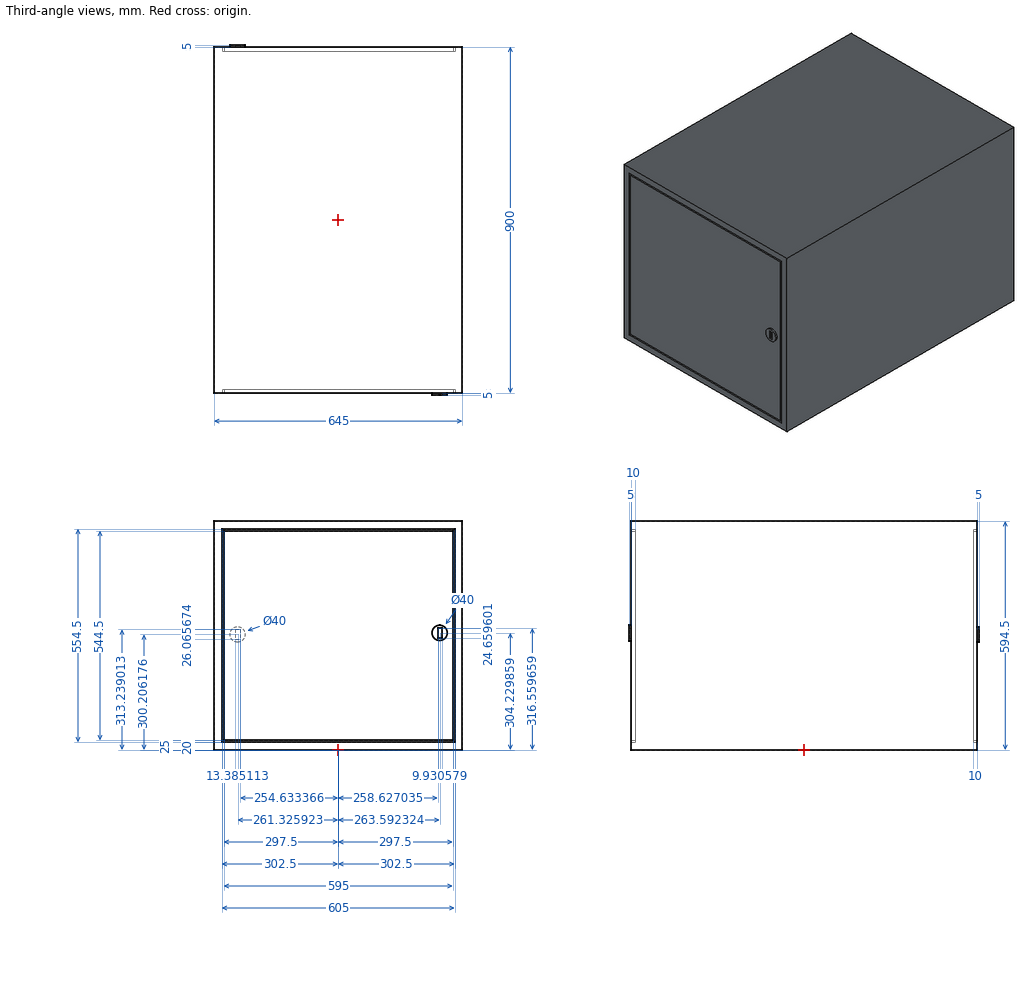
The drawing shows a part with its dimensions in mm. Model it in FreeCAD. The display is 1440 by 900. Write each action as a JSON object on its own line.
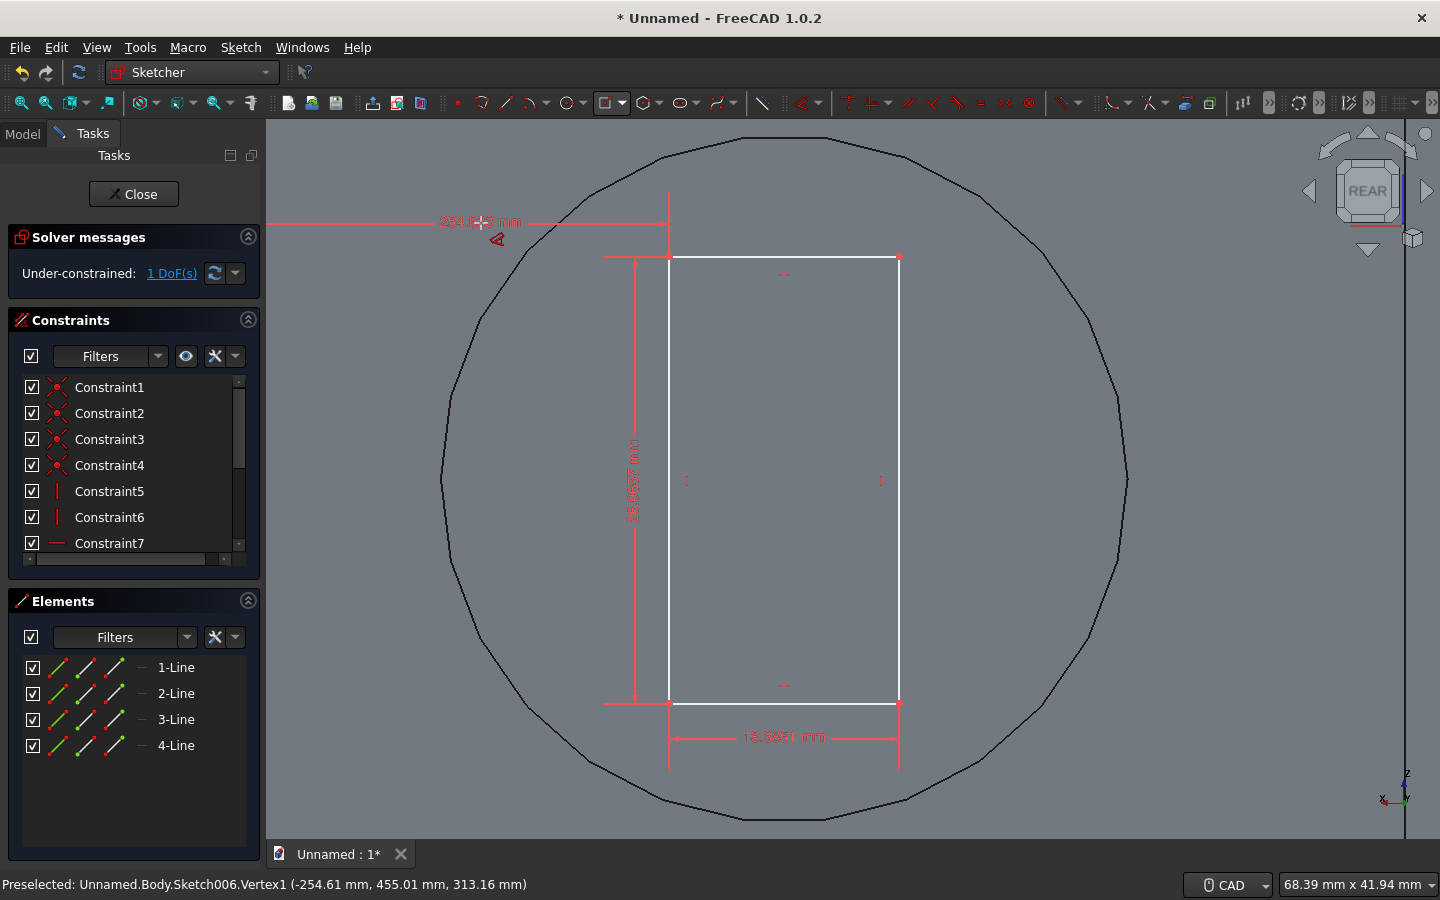
{"action": "left_click", "coordinate": [669, 257]}
{"action": "left_click", "coordinate": [703, 534]}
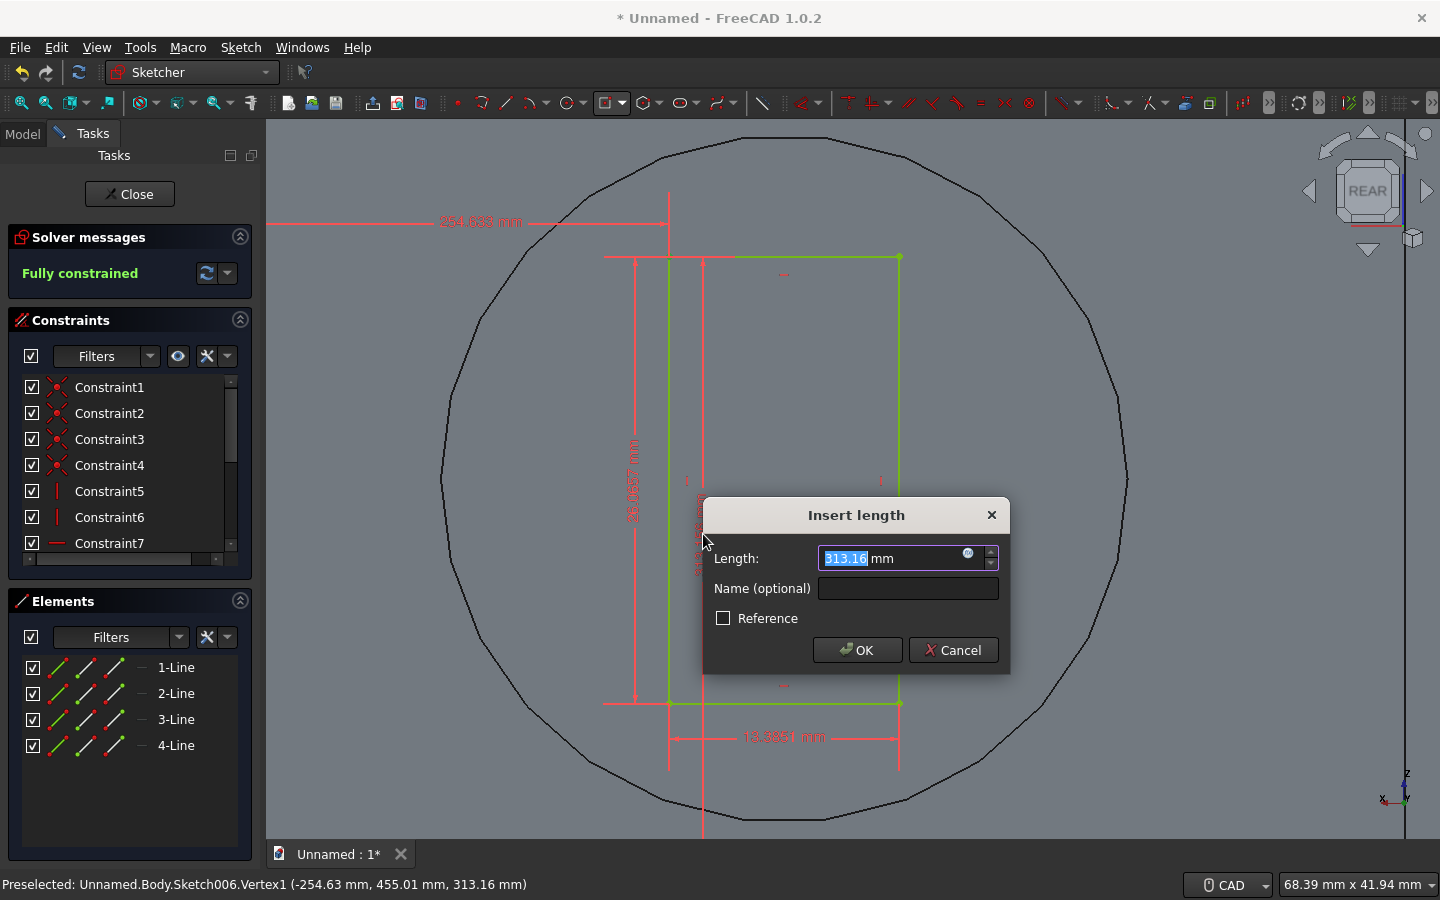
{"action": "type", "text": "313.239013"}
{"action": "key", "text": "Return"}
{"action": "key", "text": "Escape"}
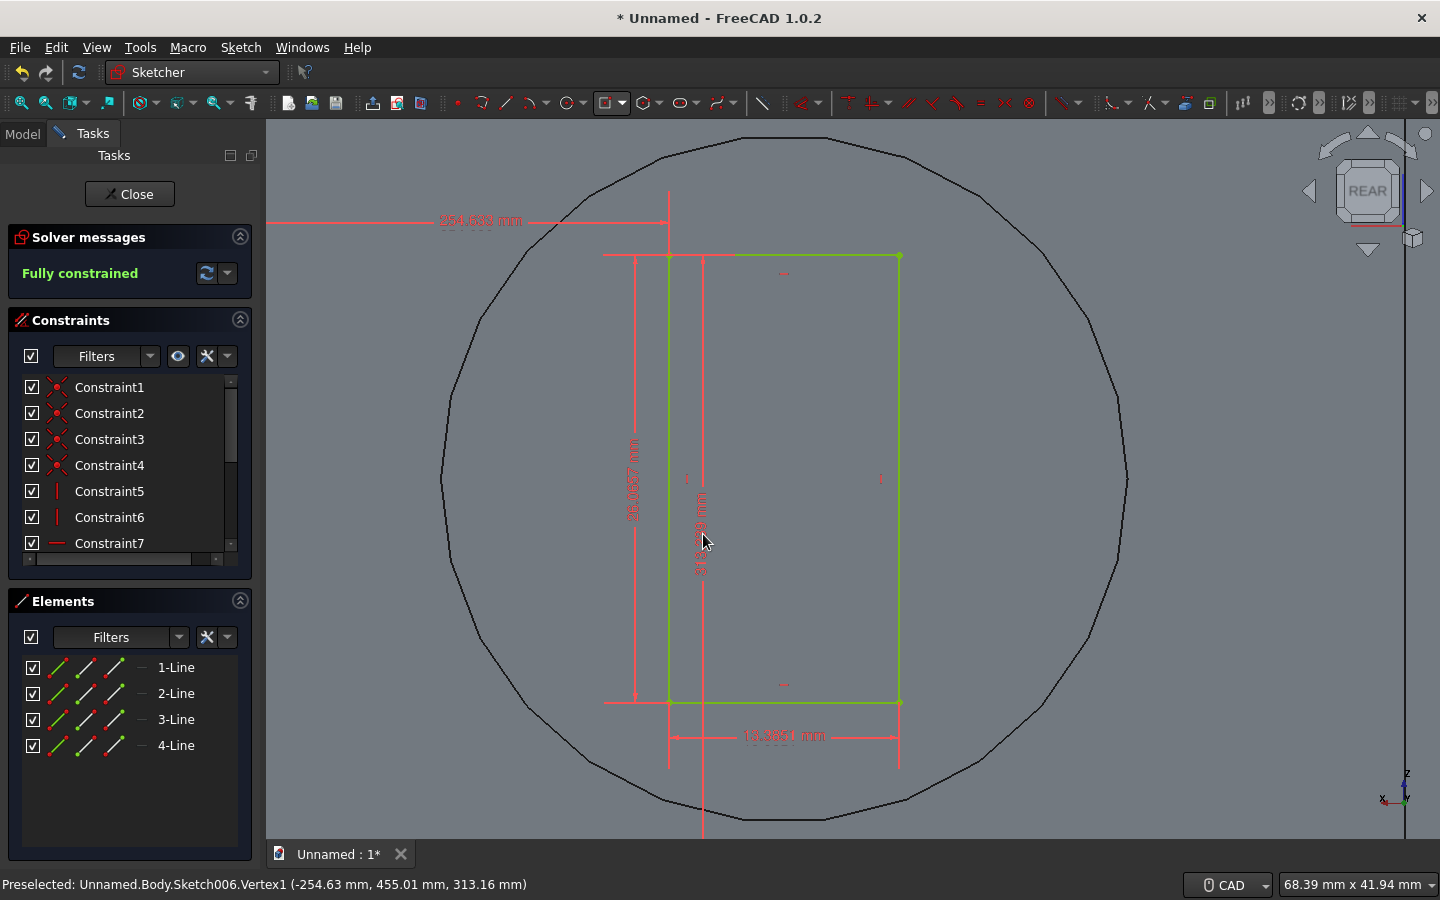
{"action": "left_click", "coordinate": [130, 194]}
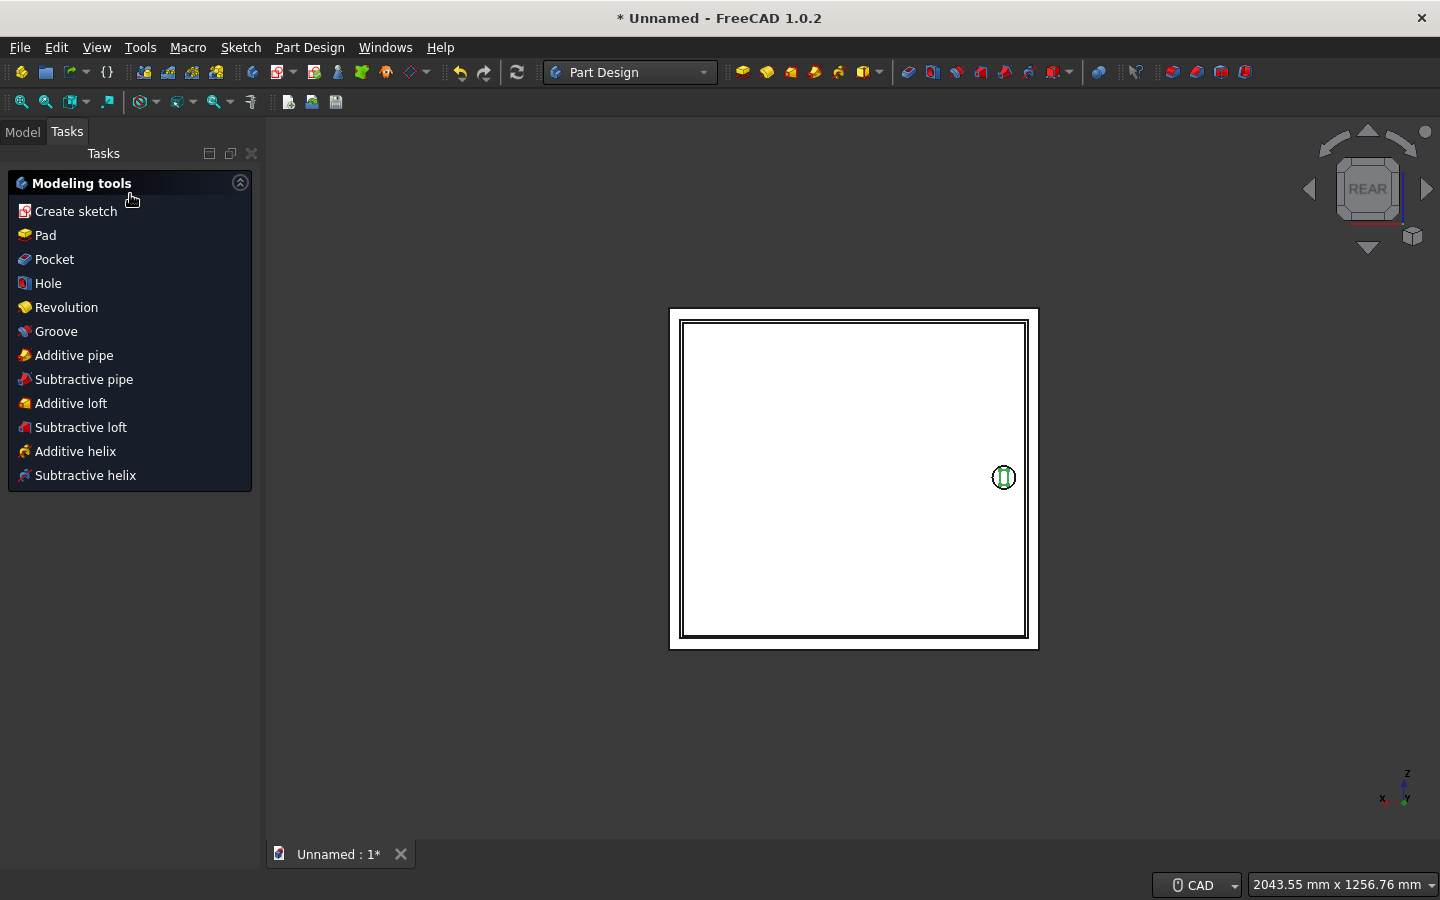
{"action": "left_click", "coordinate": [910, 72]}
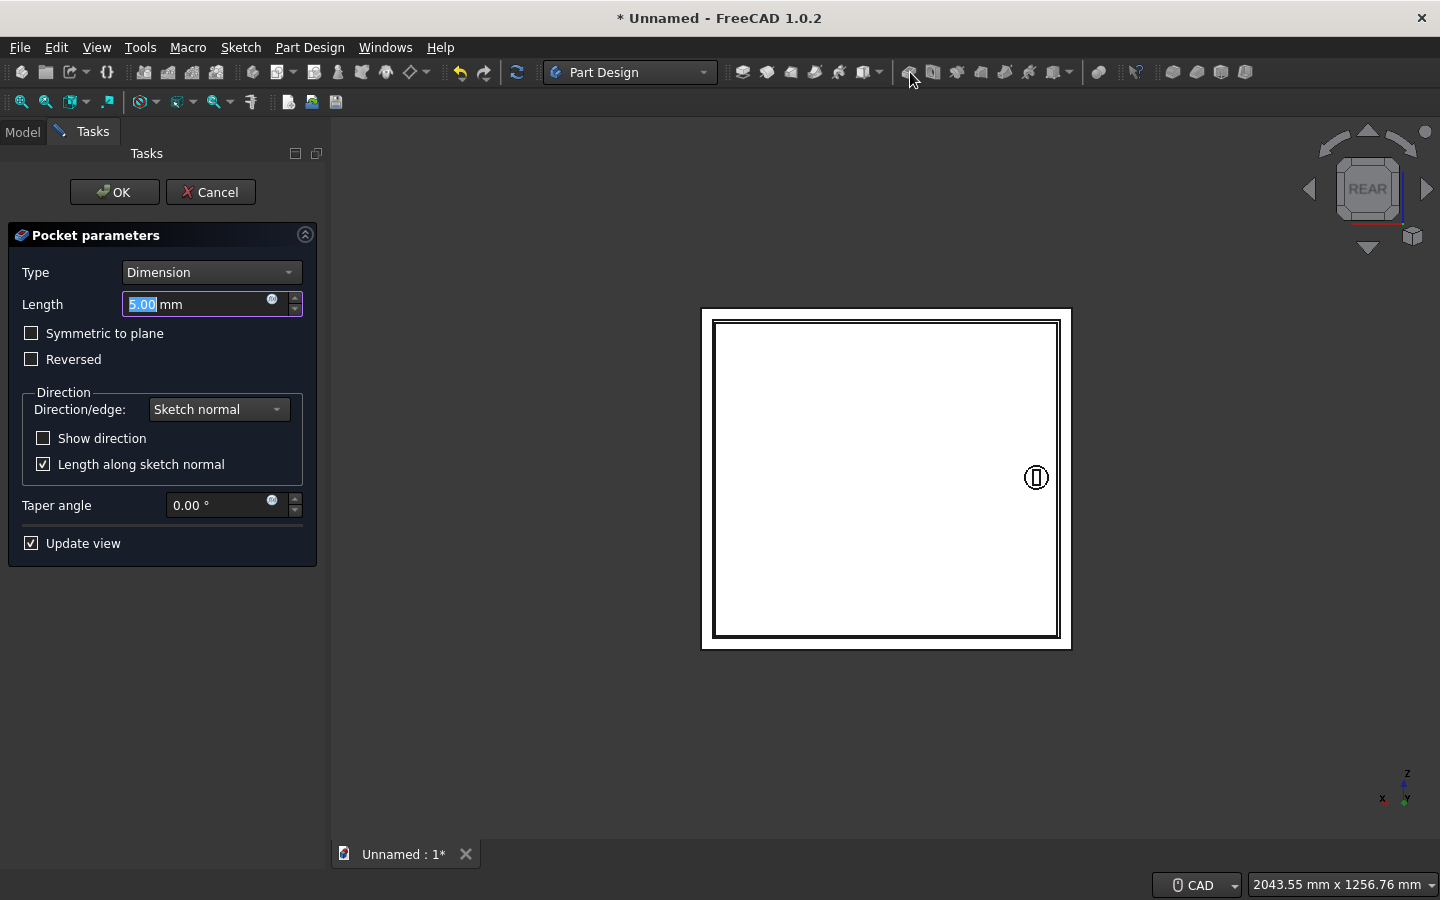
{"action": "type", "text": "5"}
{"action": "key", "text": "Tab"}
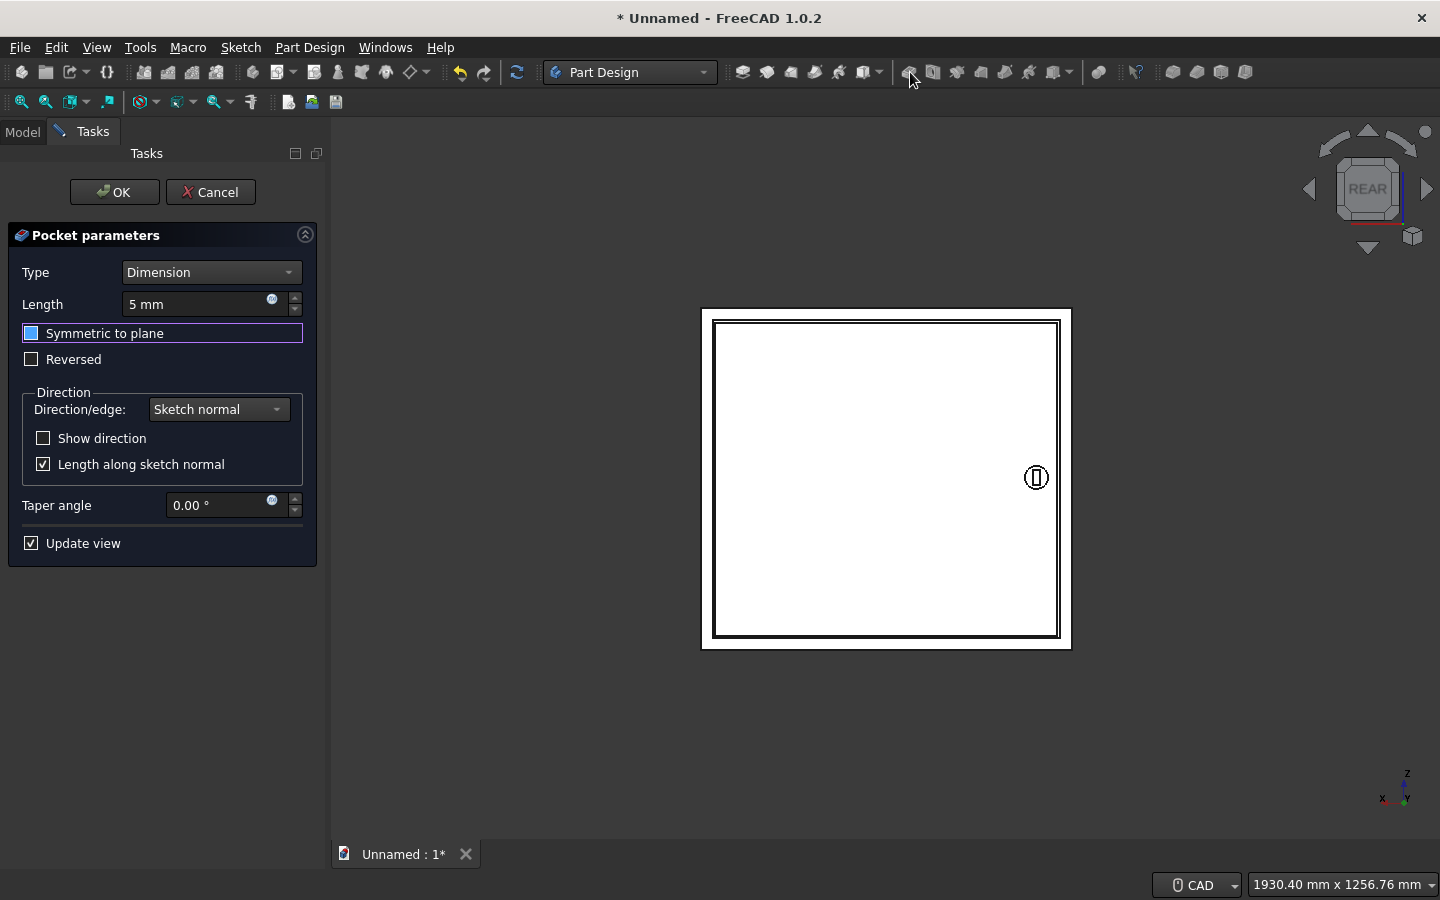
{"action": "left_click", "coordinate": [115, 192]}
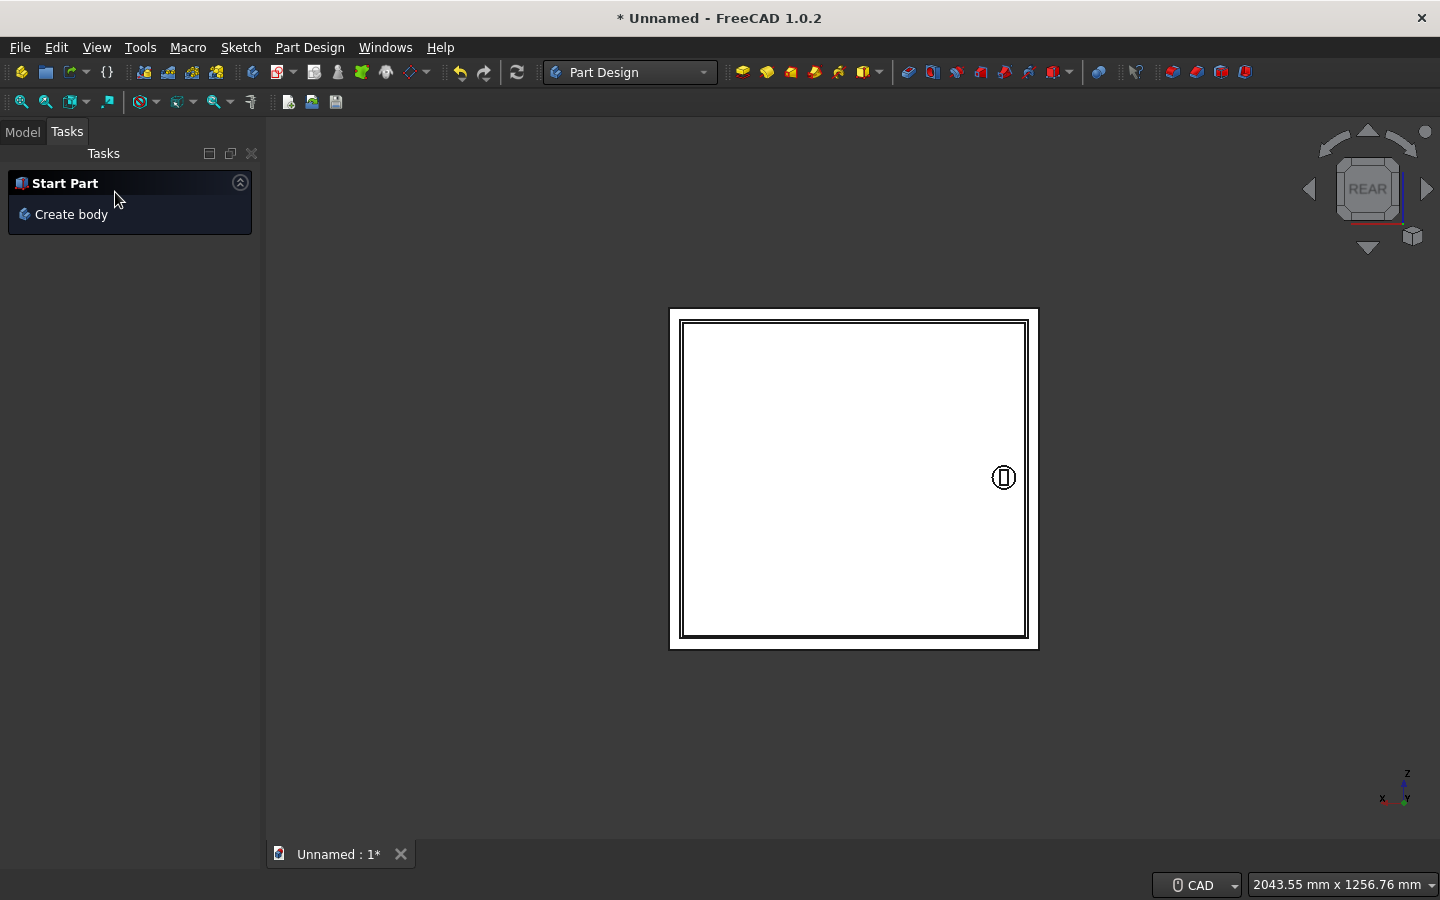
{"action": "key", "text": "0"}